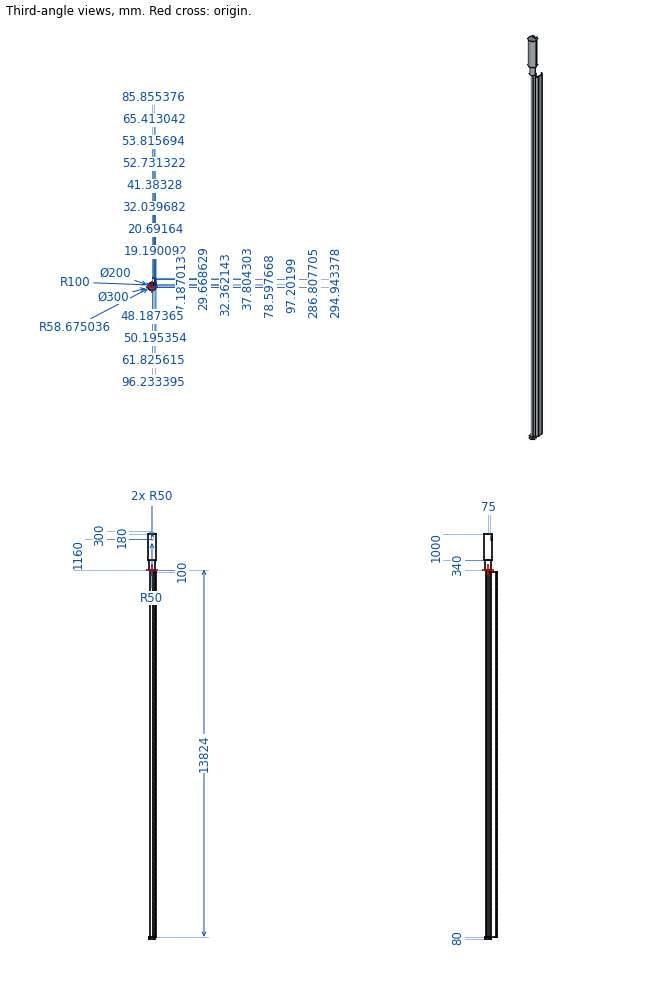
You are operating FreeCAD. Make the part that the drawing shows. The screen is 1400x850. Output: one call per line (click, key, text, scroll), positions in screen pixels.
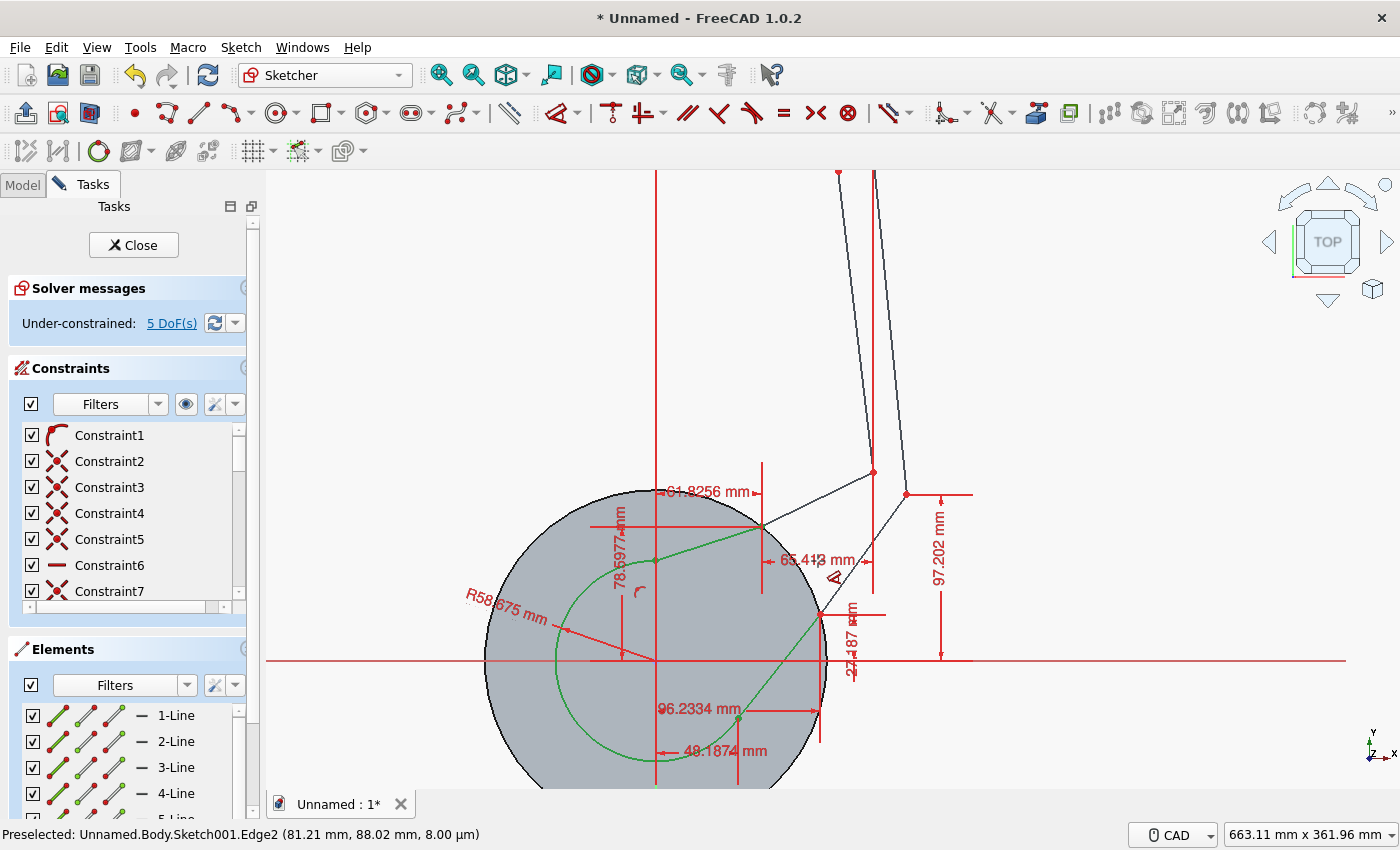
click(795, 510)
click(907, 518)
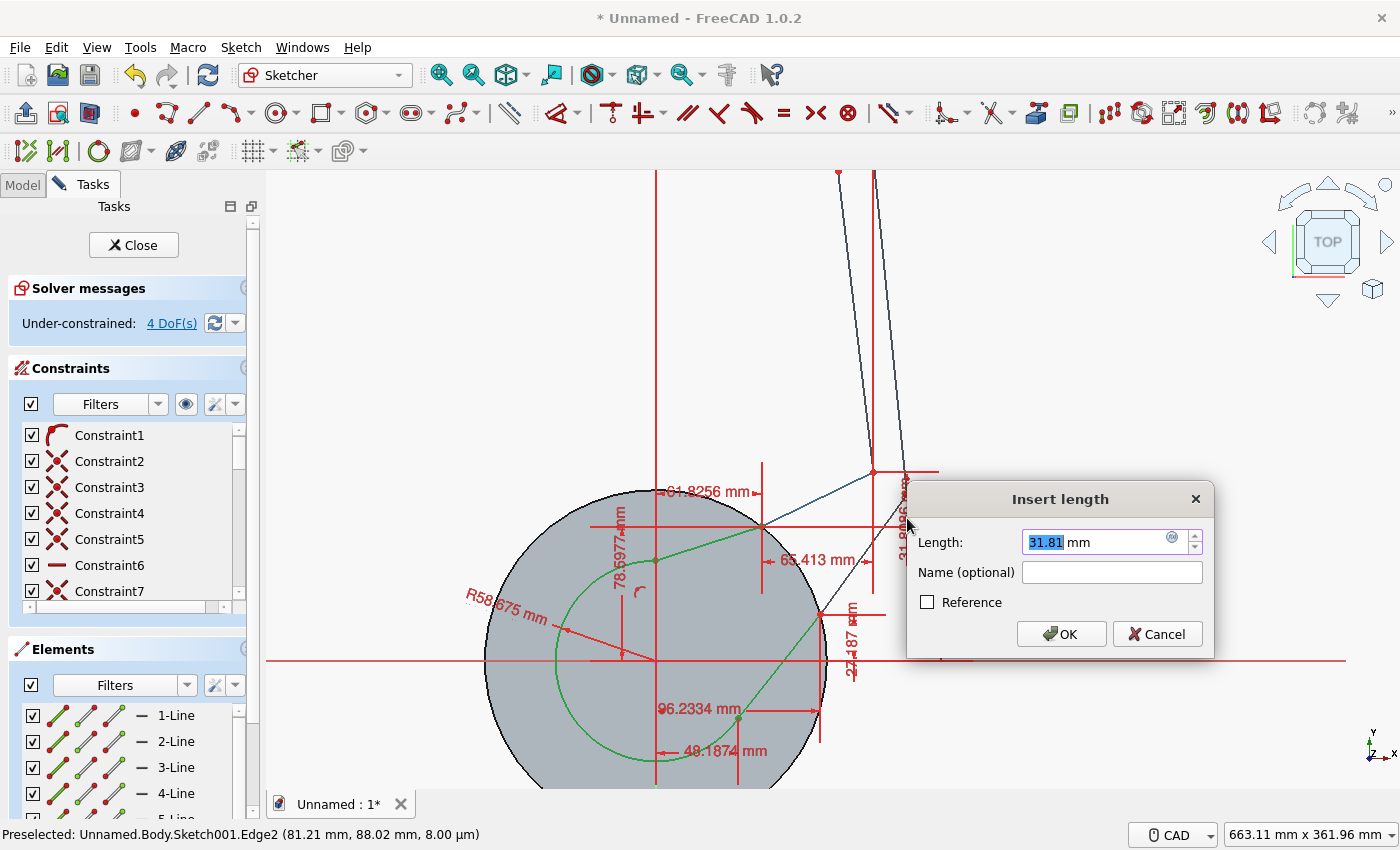
text(32.362143)
key(Return)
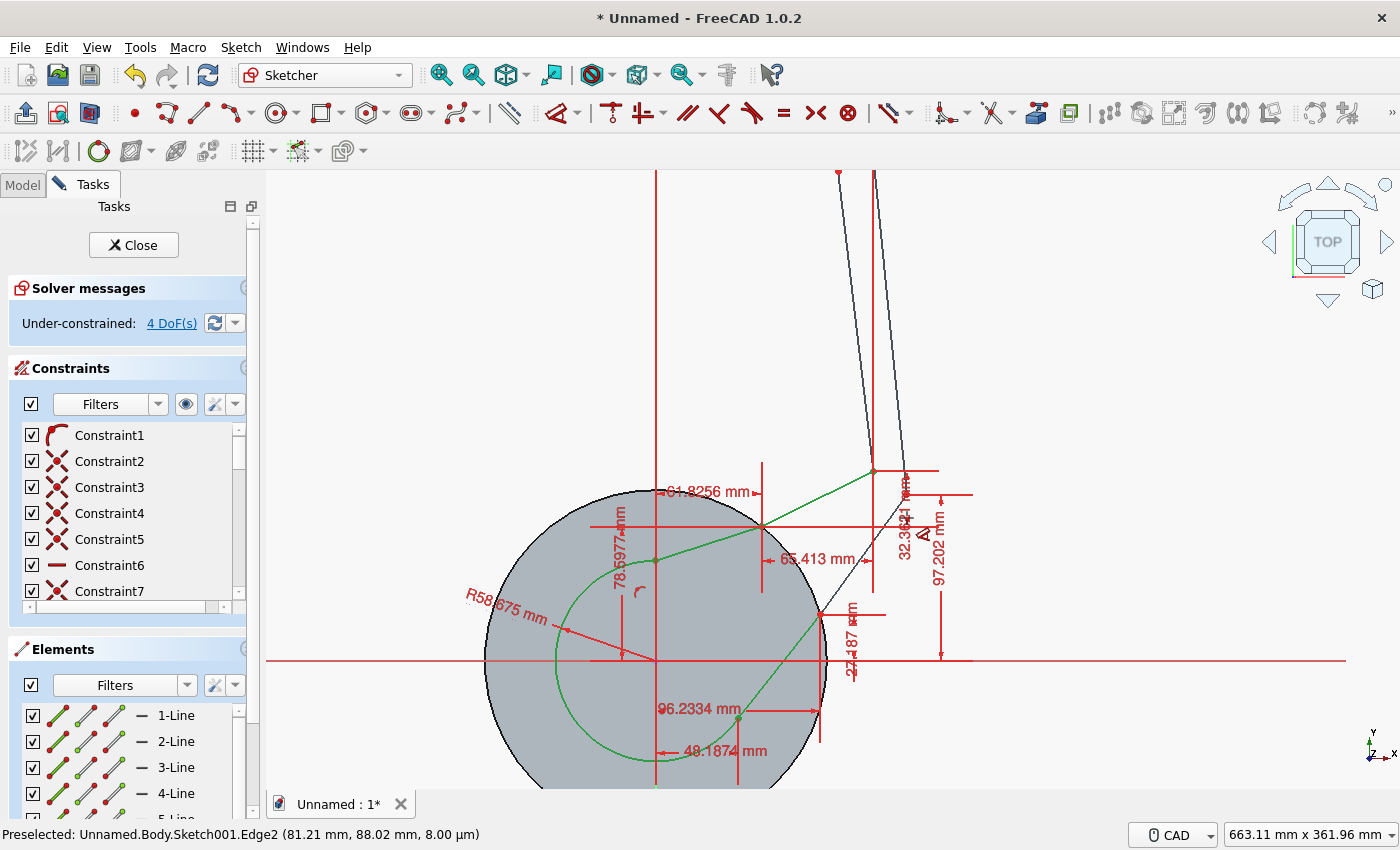
scroll(821, 617, down, 2)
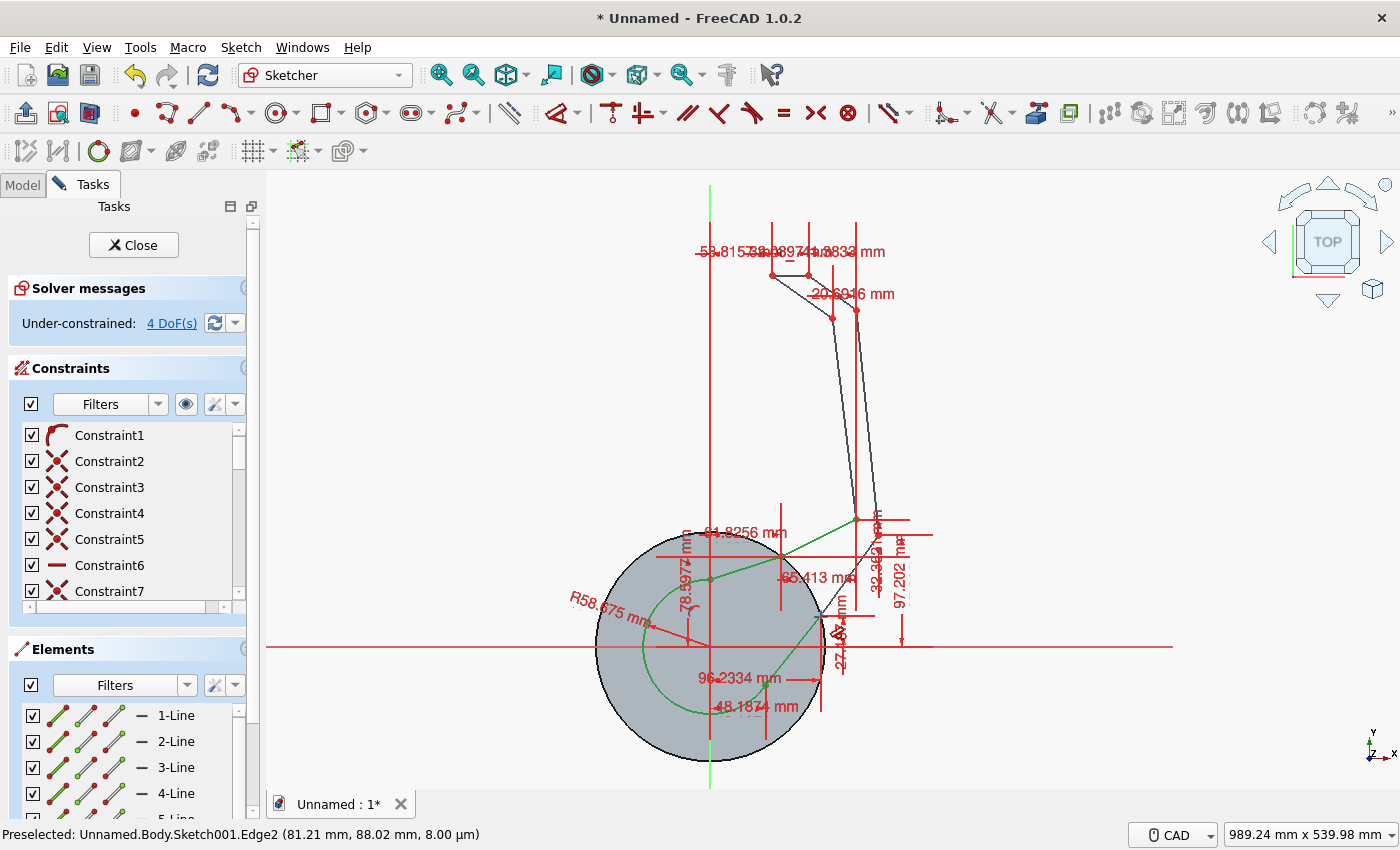
click(814, 306)
click(738, 297)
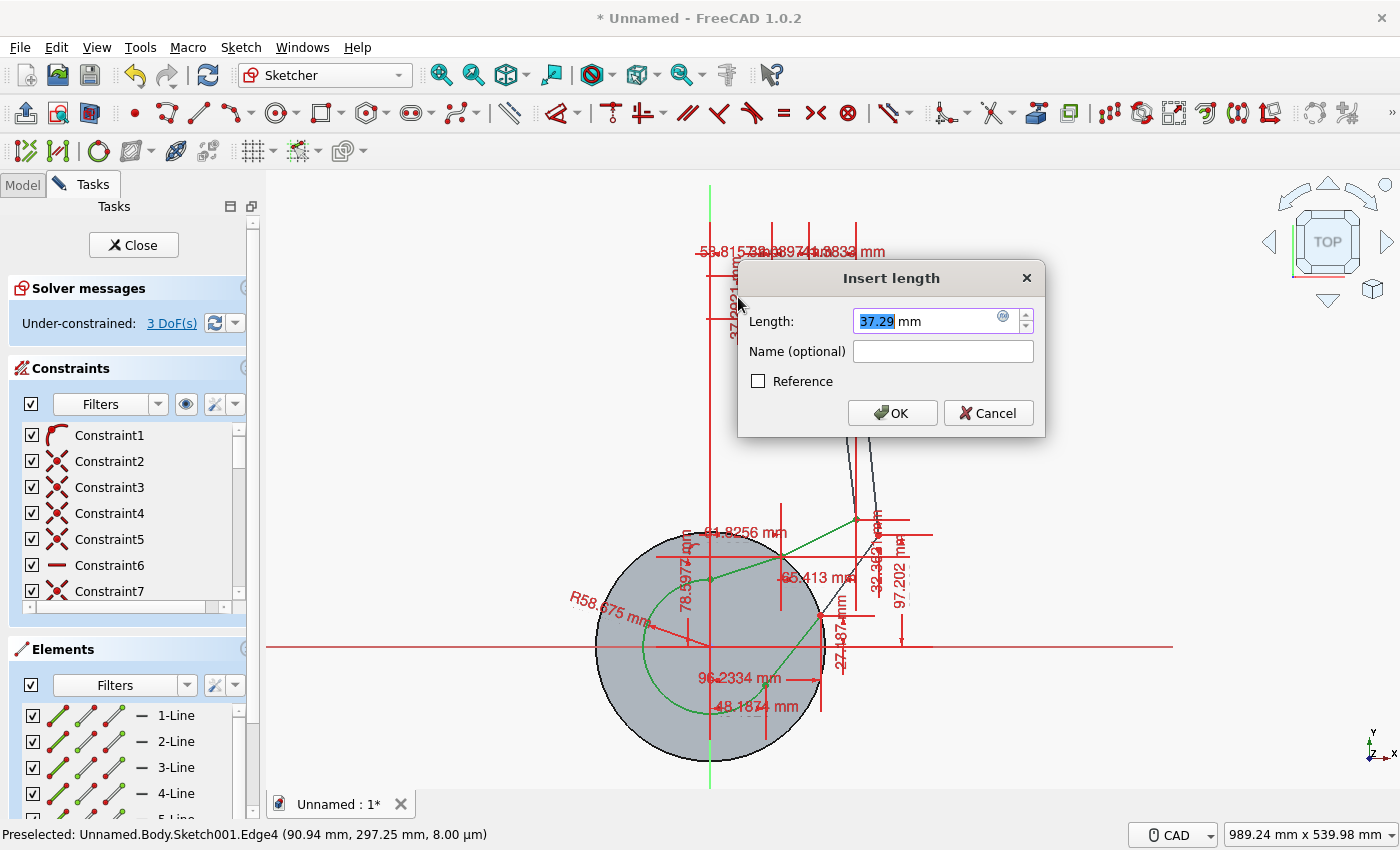
text(37.804303)
key(Return)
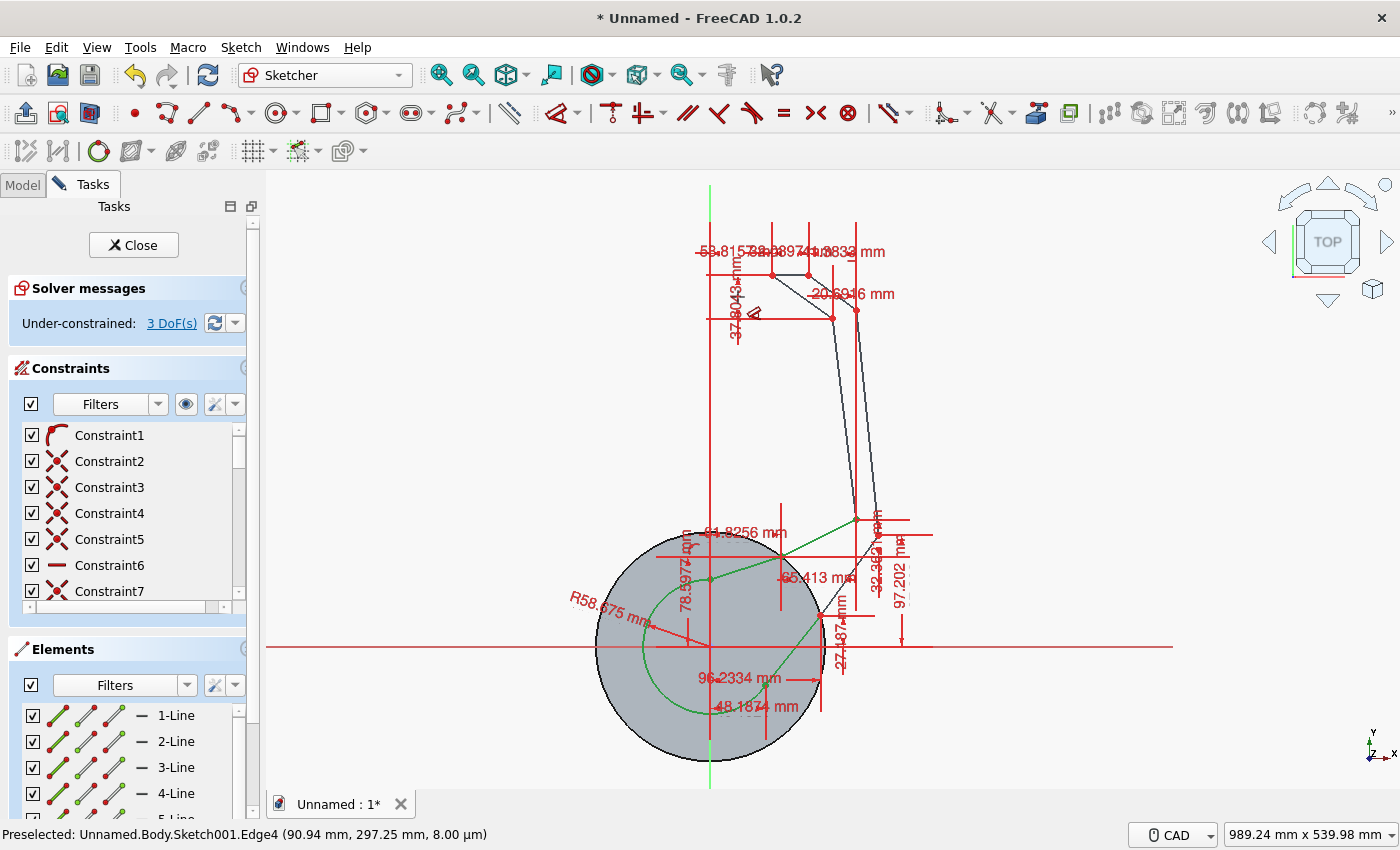
click(823, 286)
click(938, 293)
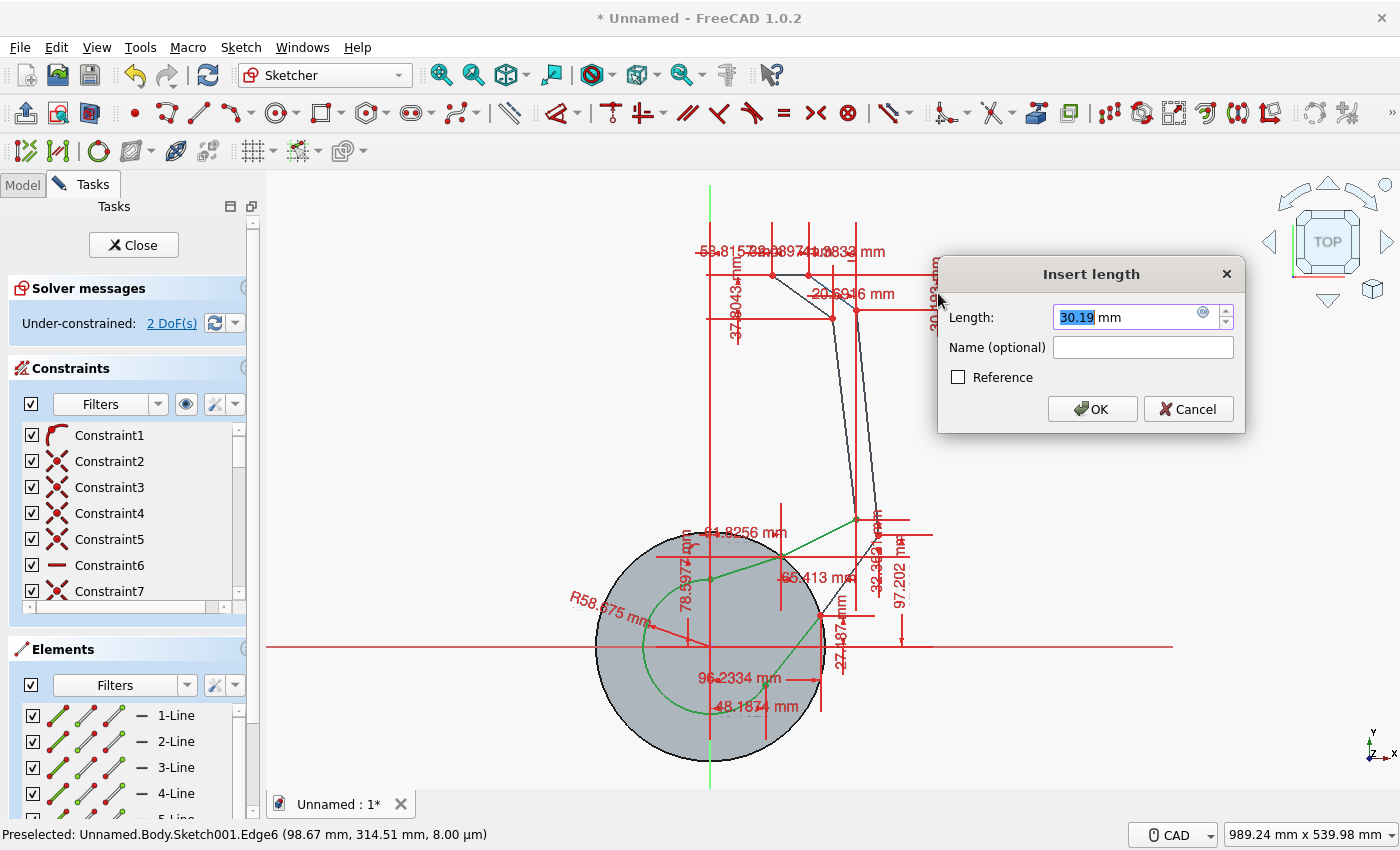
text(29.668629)
key(Return)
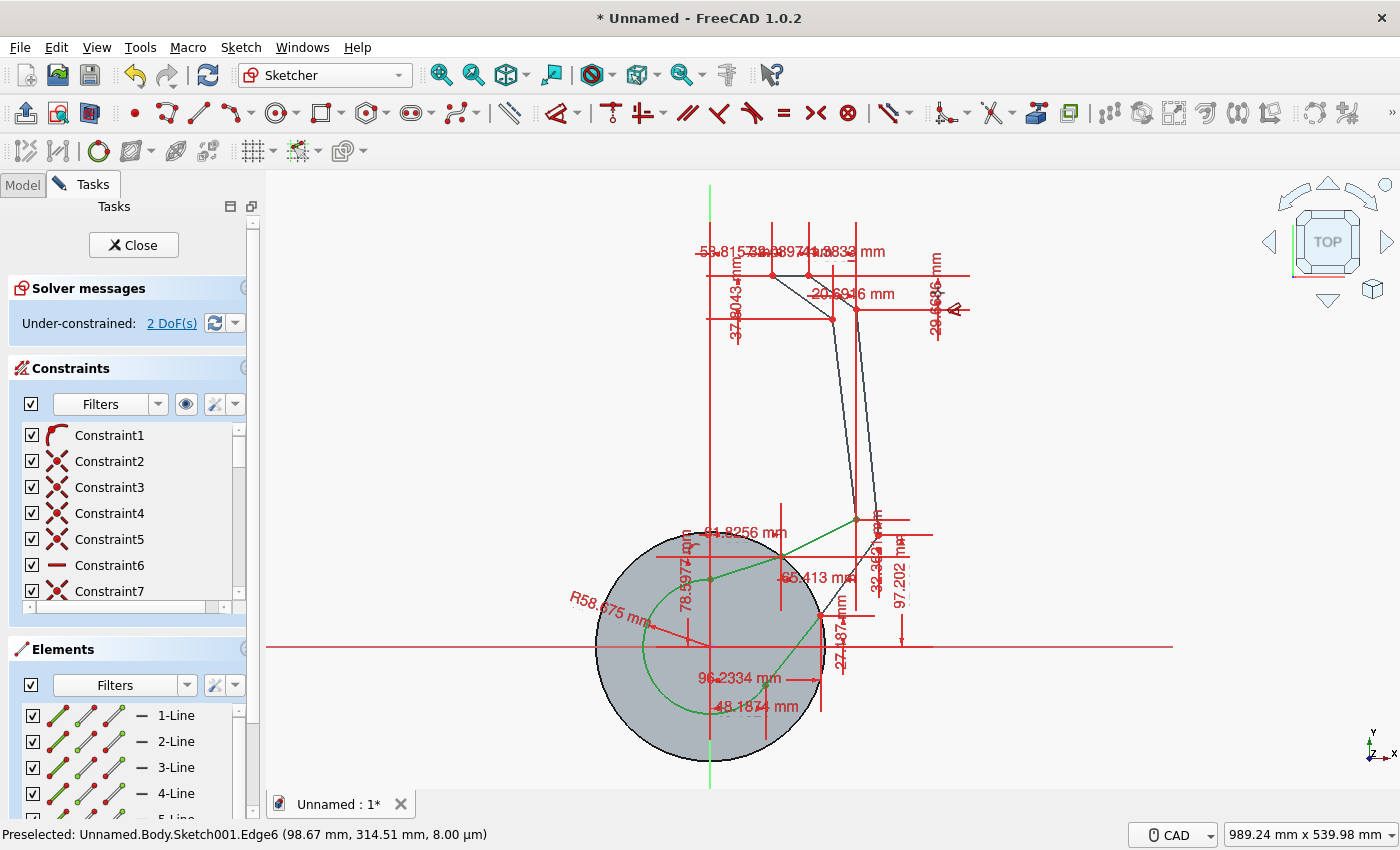
scroll(863, 378, up, 3)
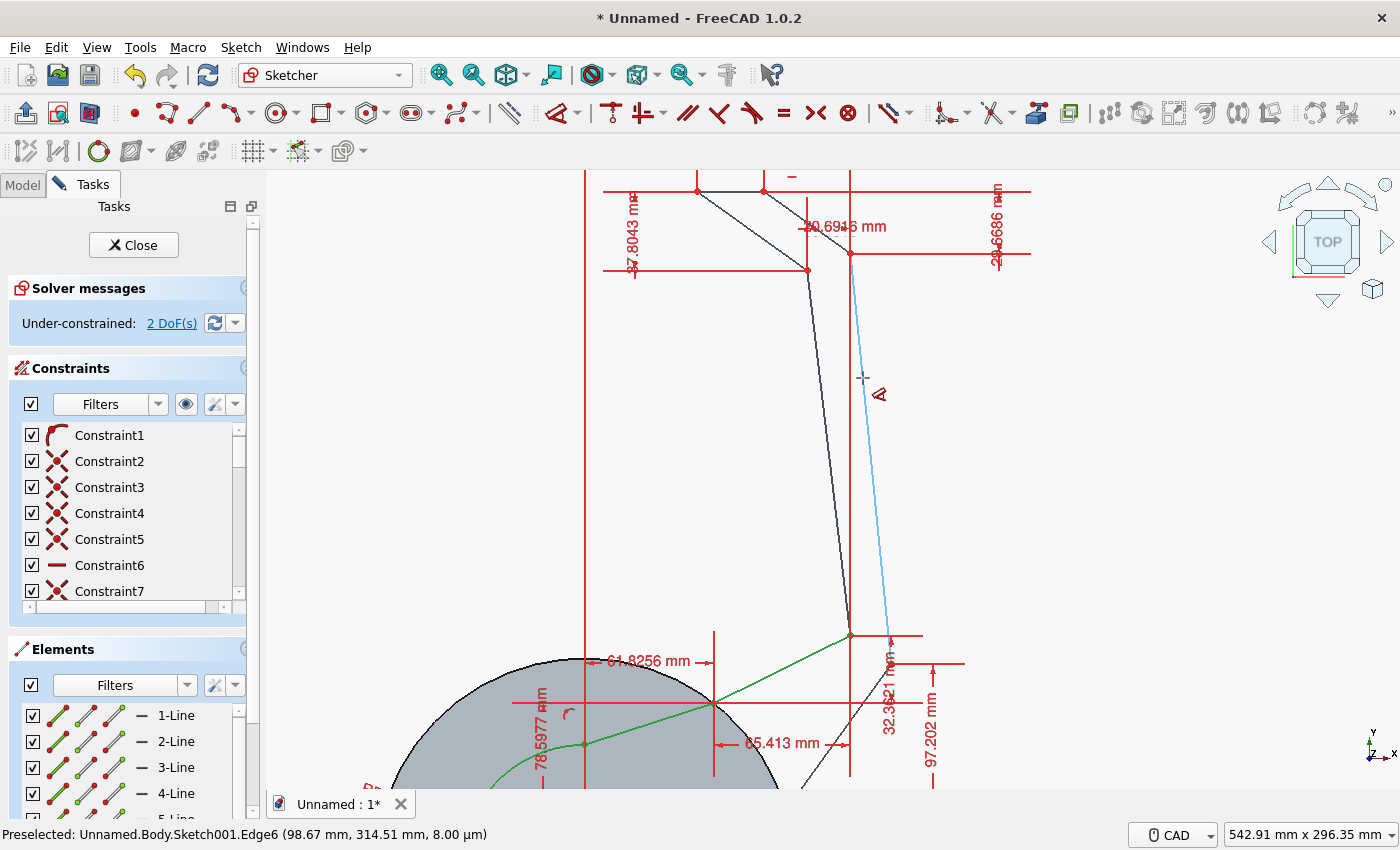
click(863, 377)
click(861, 746)